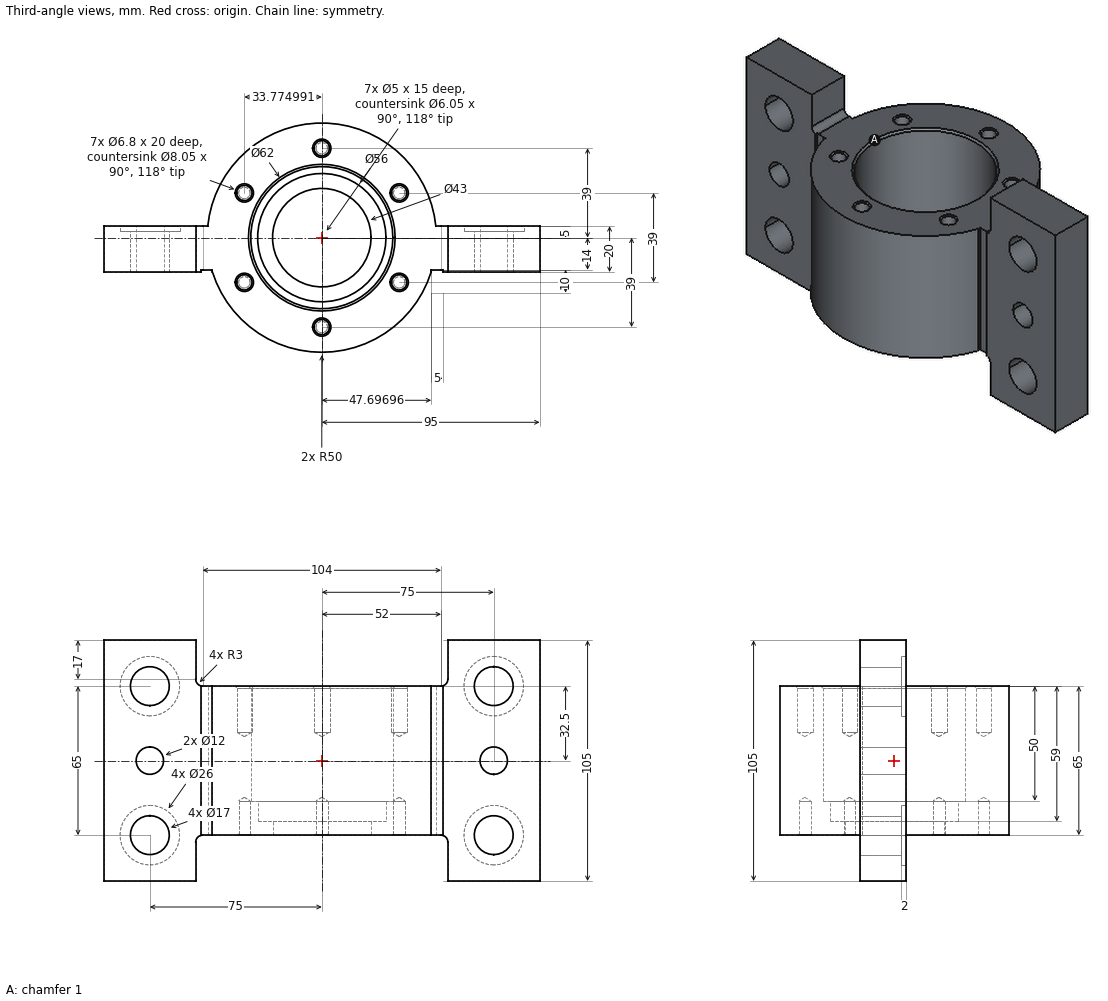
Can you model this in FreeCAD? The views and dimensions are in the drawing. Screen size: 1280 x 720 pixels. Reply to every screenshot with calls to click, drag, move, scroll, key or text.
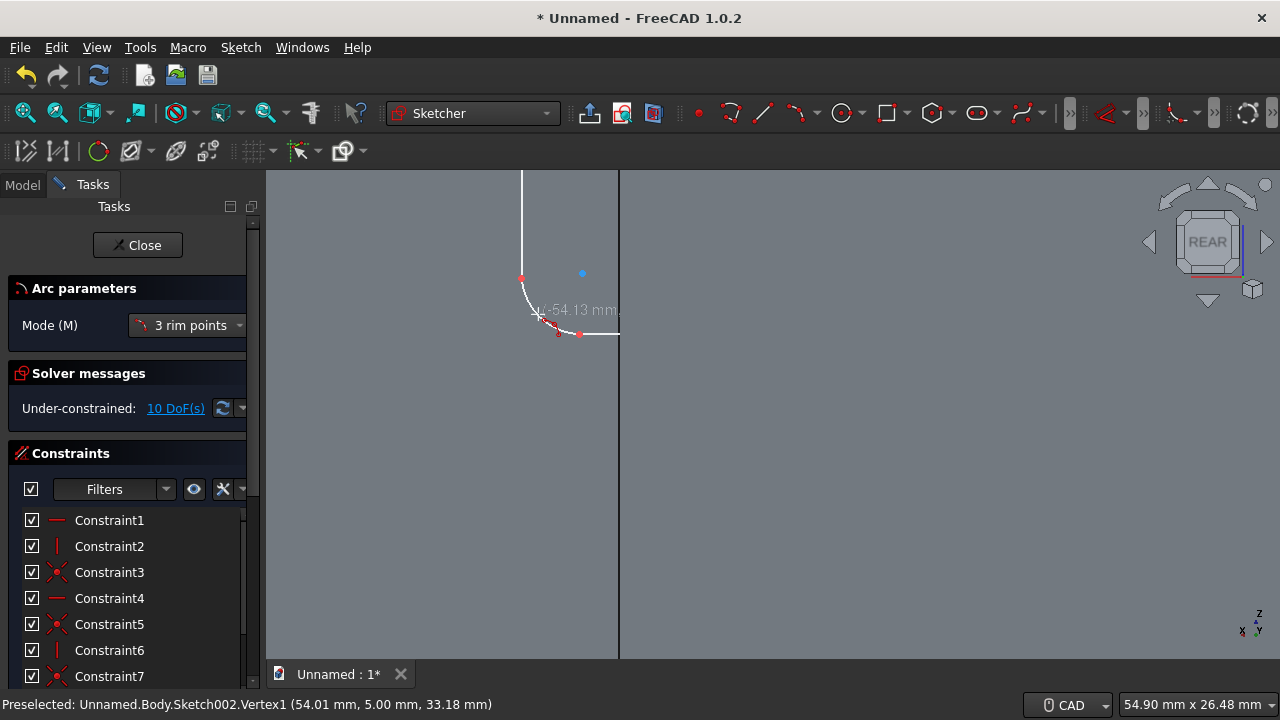
click(764, 114)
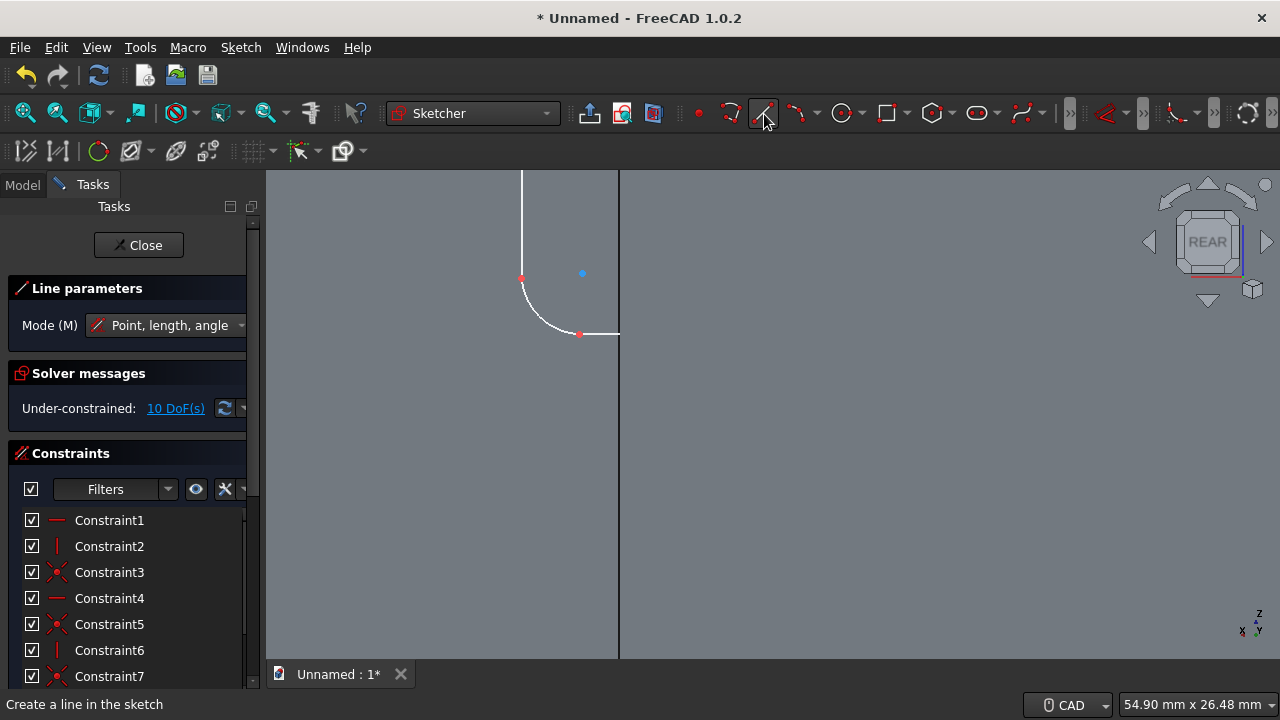
scroll(539, 312, down, 9)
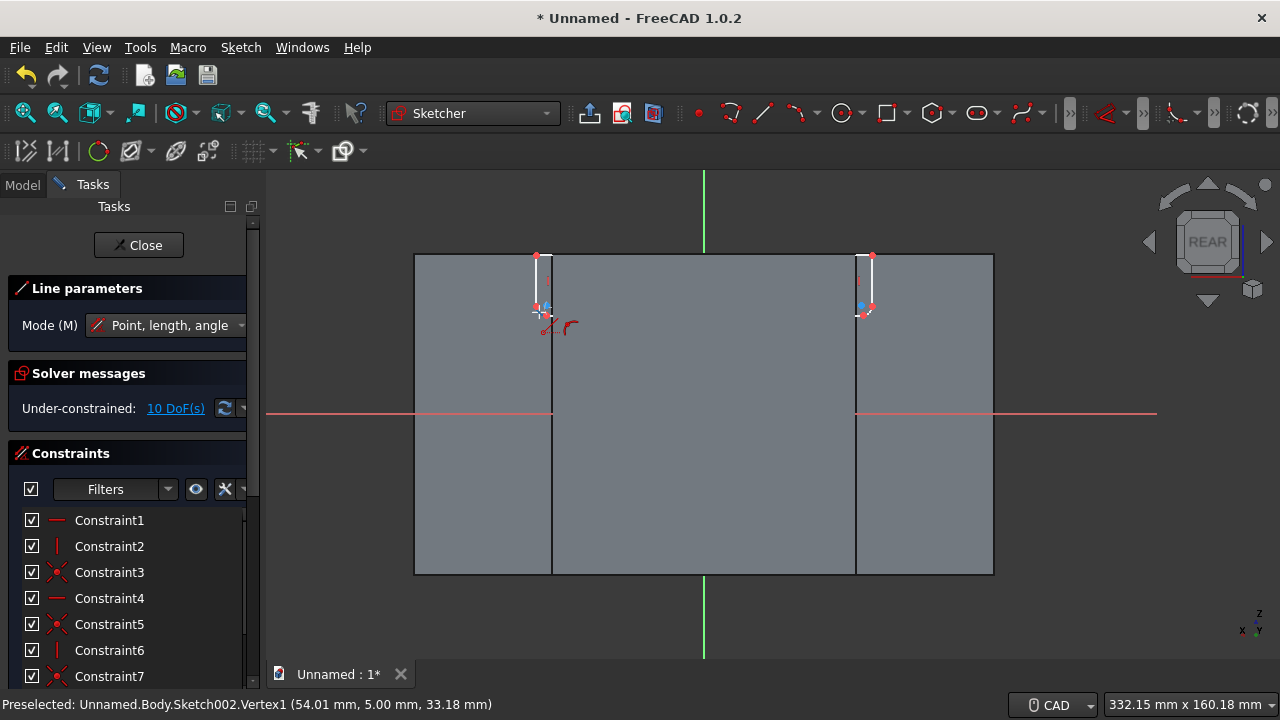
click(863, 514)
click(546, 514)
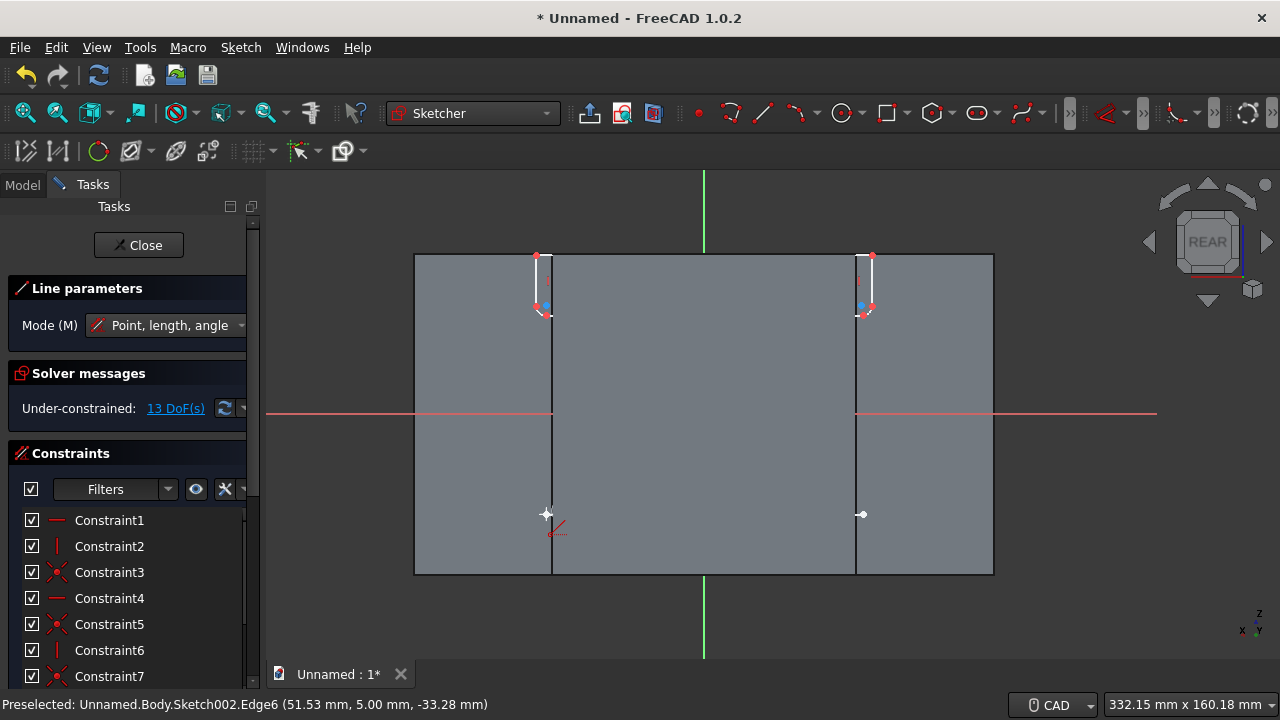
click(732, 114)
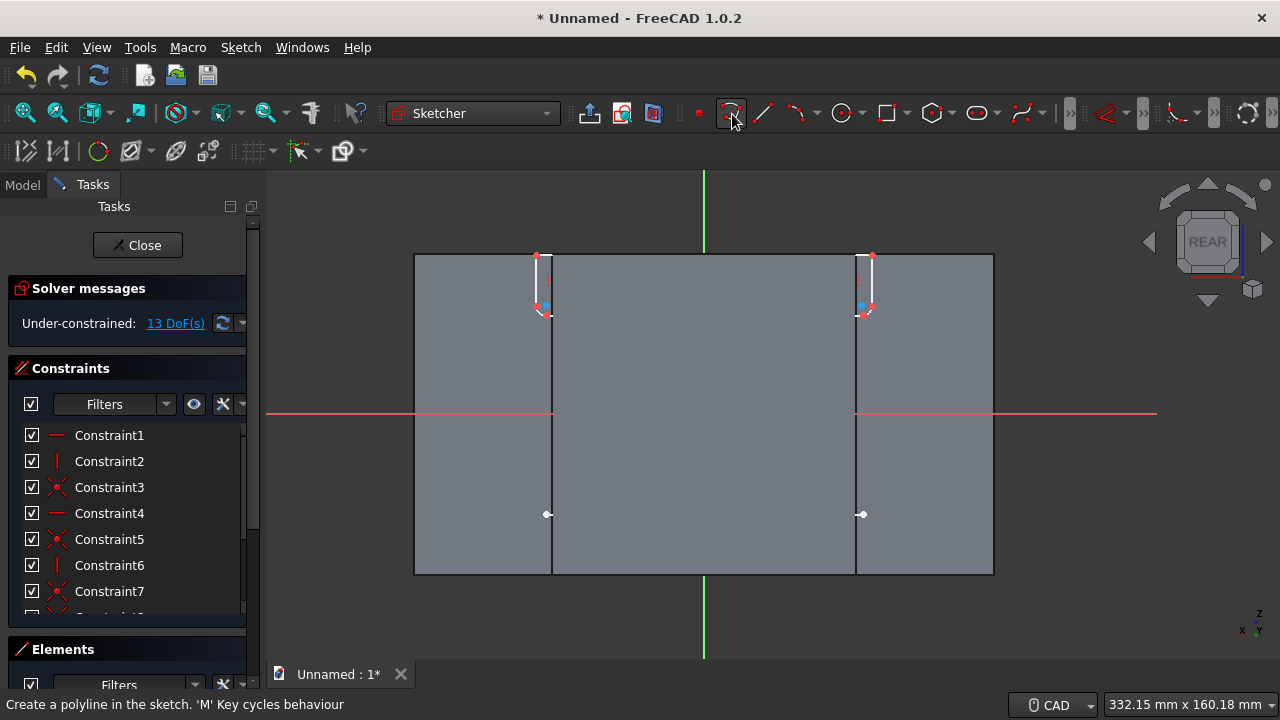
scroll(536, 523, up, 2)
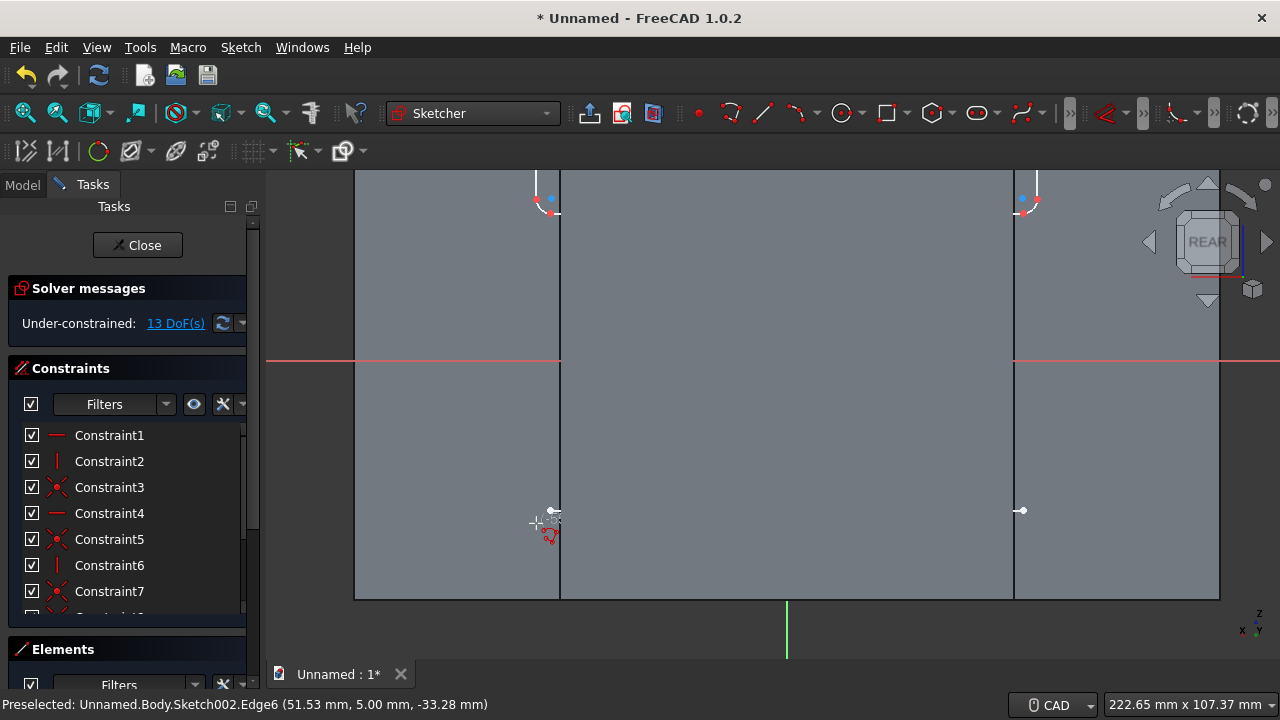
click(536, 522)
click(536, 600)
click(1037, 600)
click(1037, 522)
right_click(1037, 522)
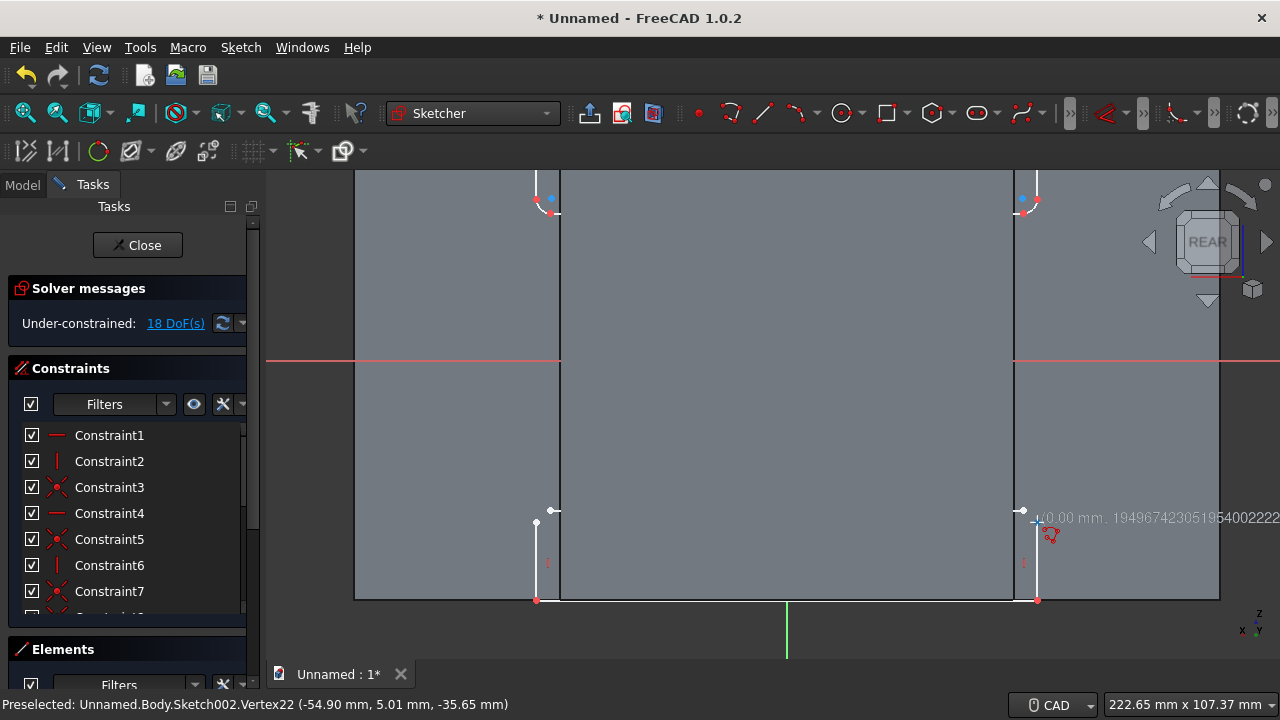
click(796, 114)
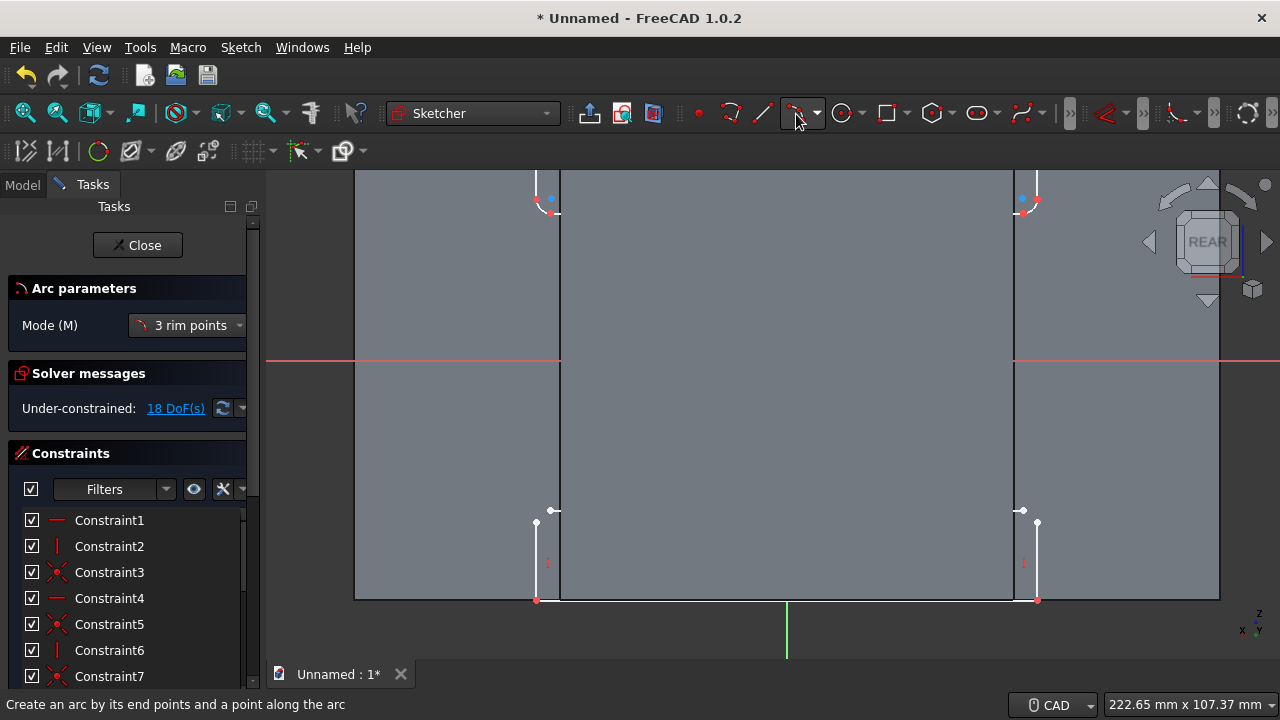
click(551, 511)
click(536, 523)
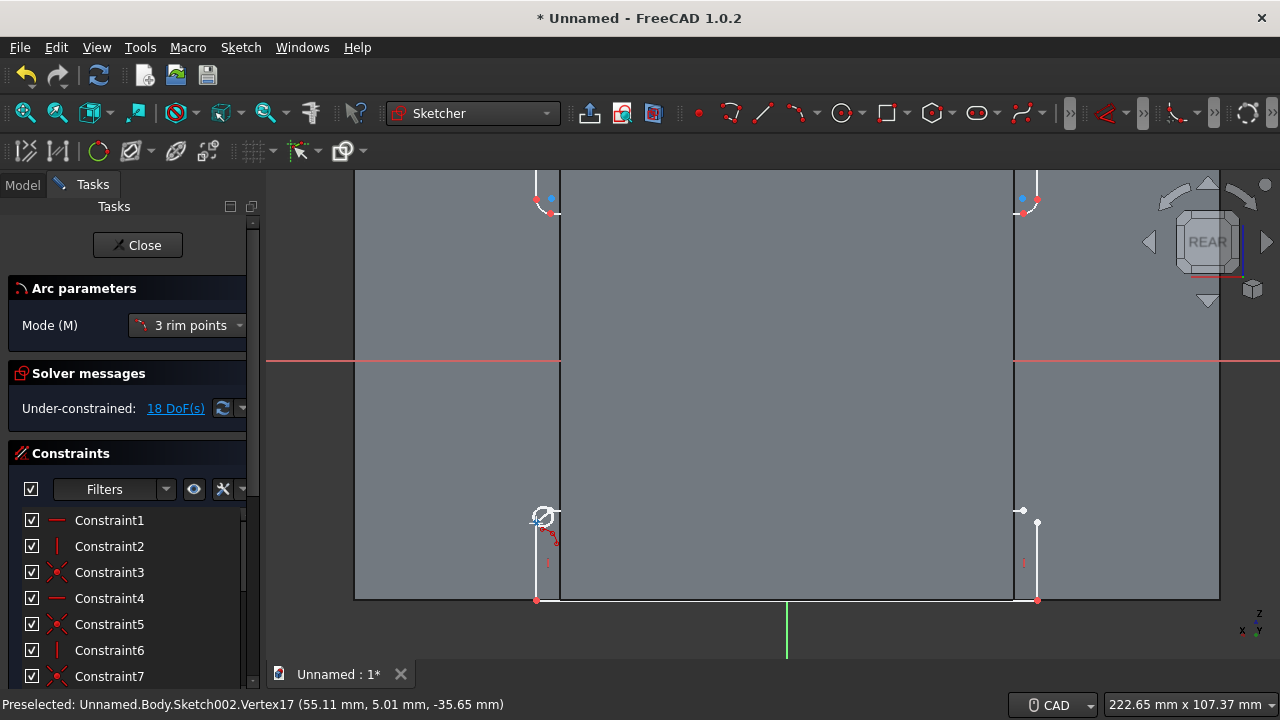
scroll(540, 513, up, 7)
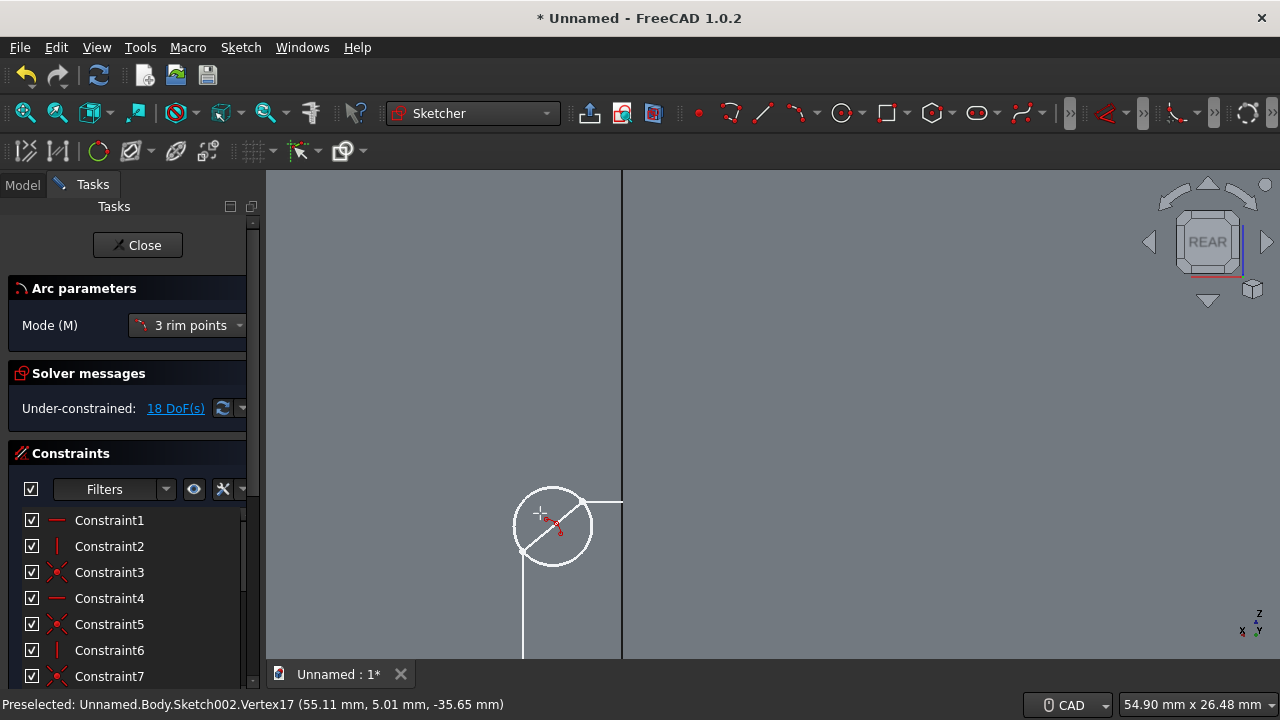
click(541, 510)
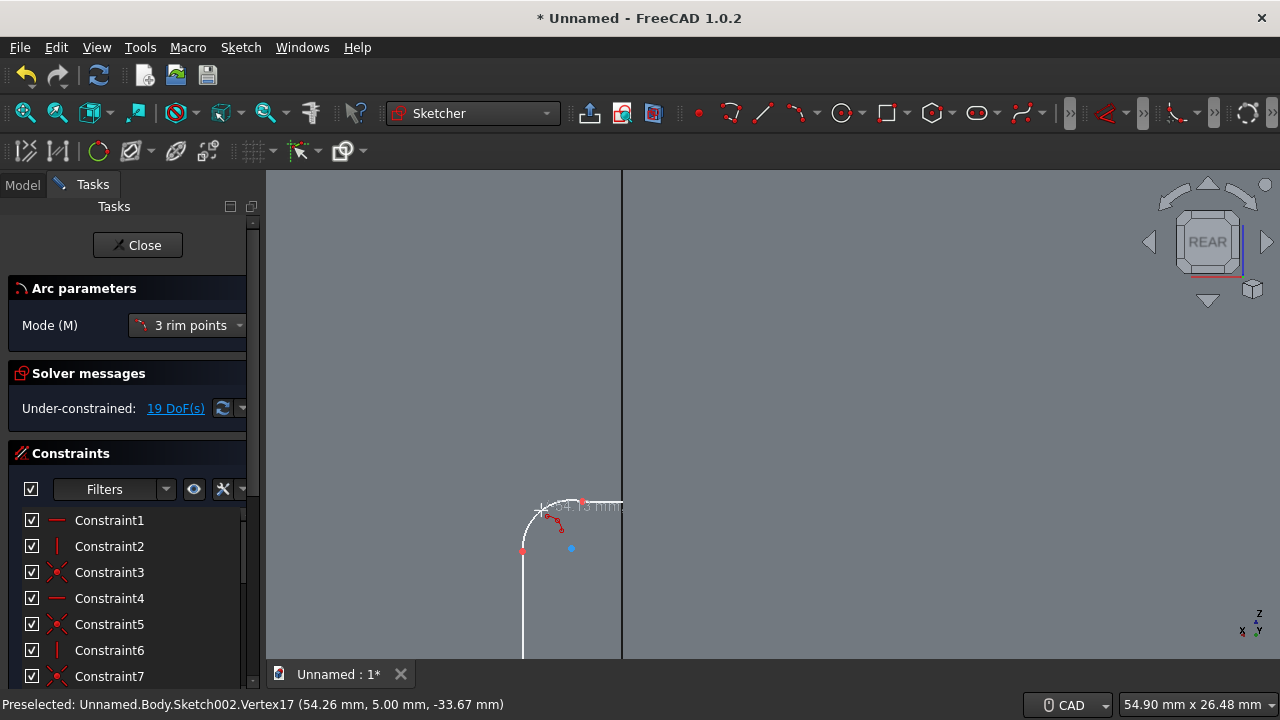
scroll(539, 518, down, 9)